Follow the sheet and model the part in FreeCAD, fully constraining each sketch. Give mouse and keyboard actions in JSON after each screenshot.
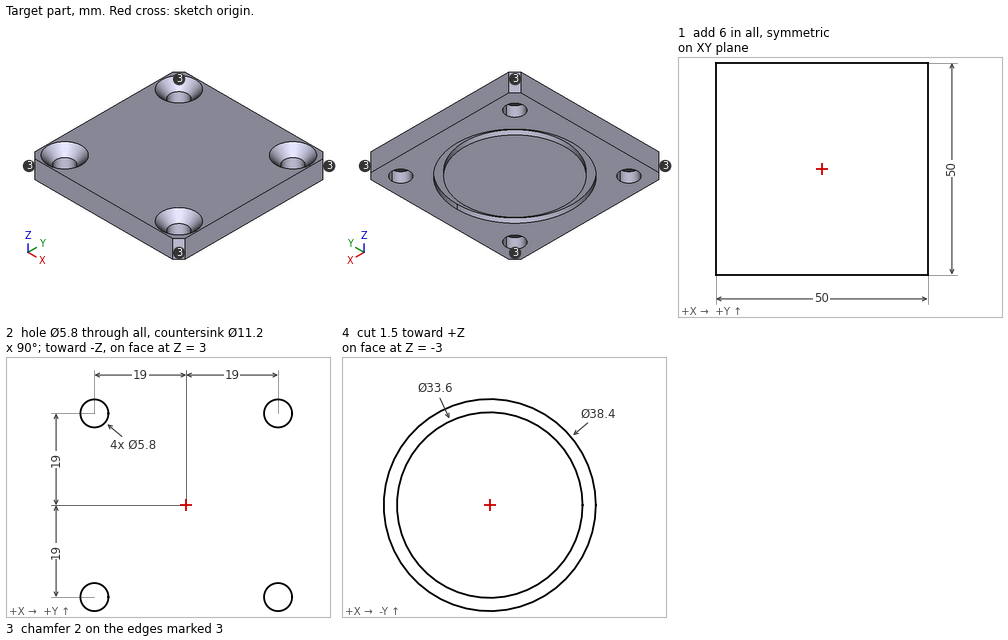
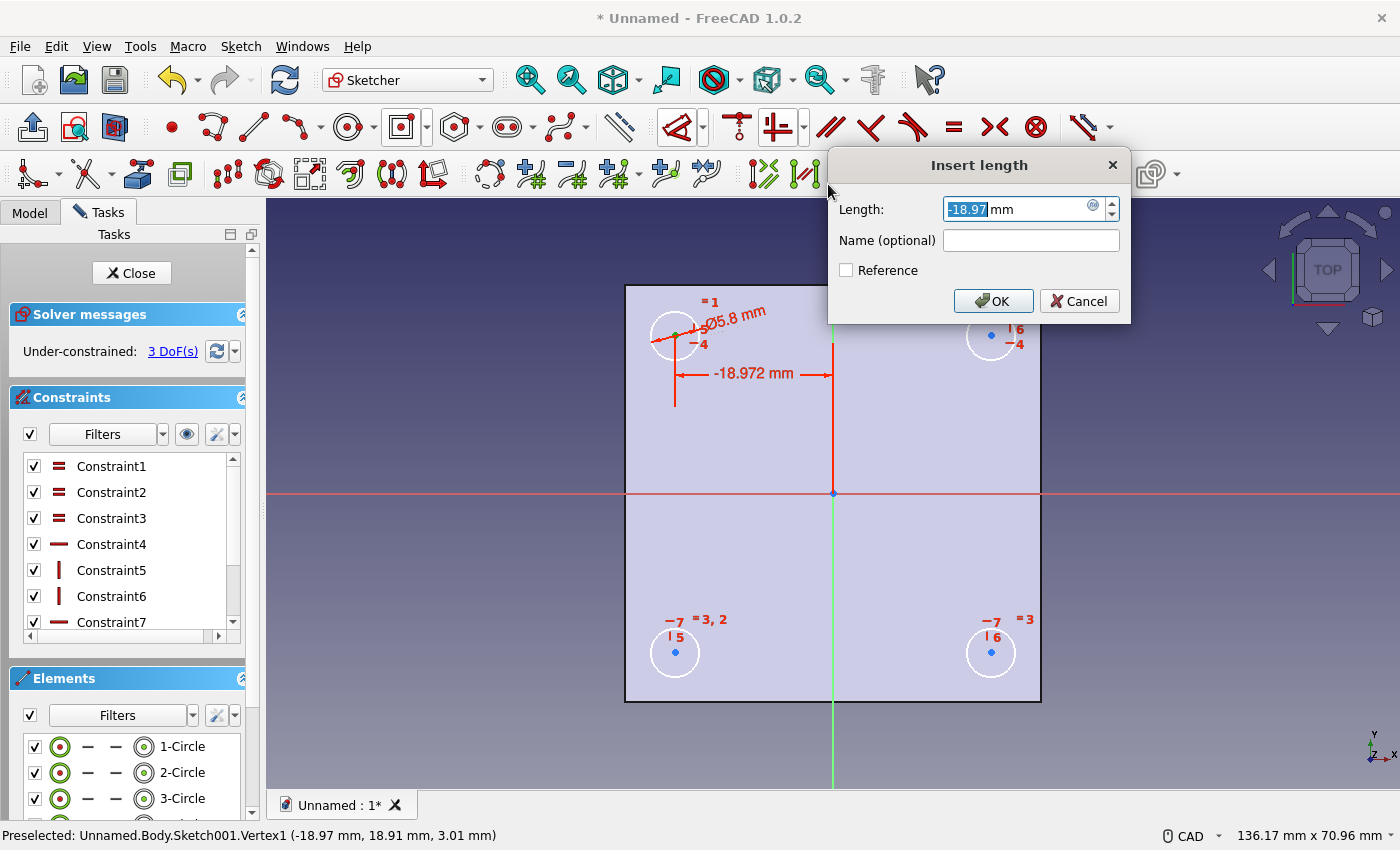
{"action": "type", "text": "-19"}
{"action": "key", "text": "Return"}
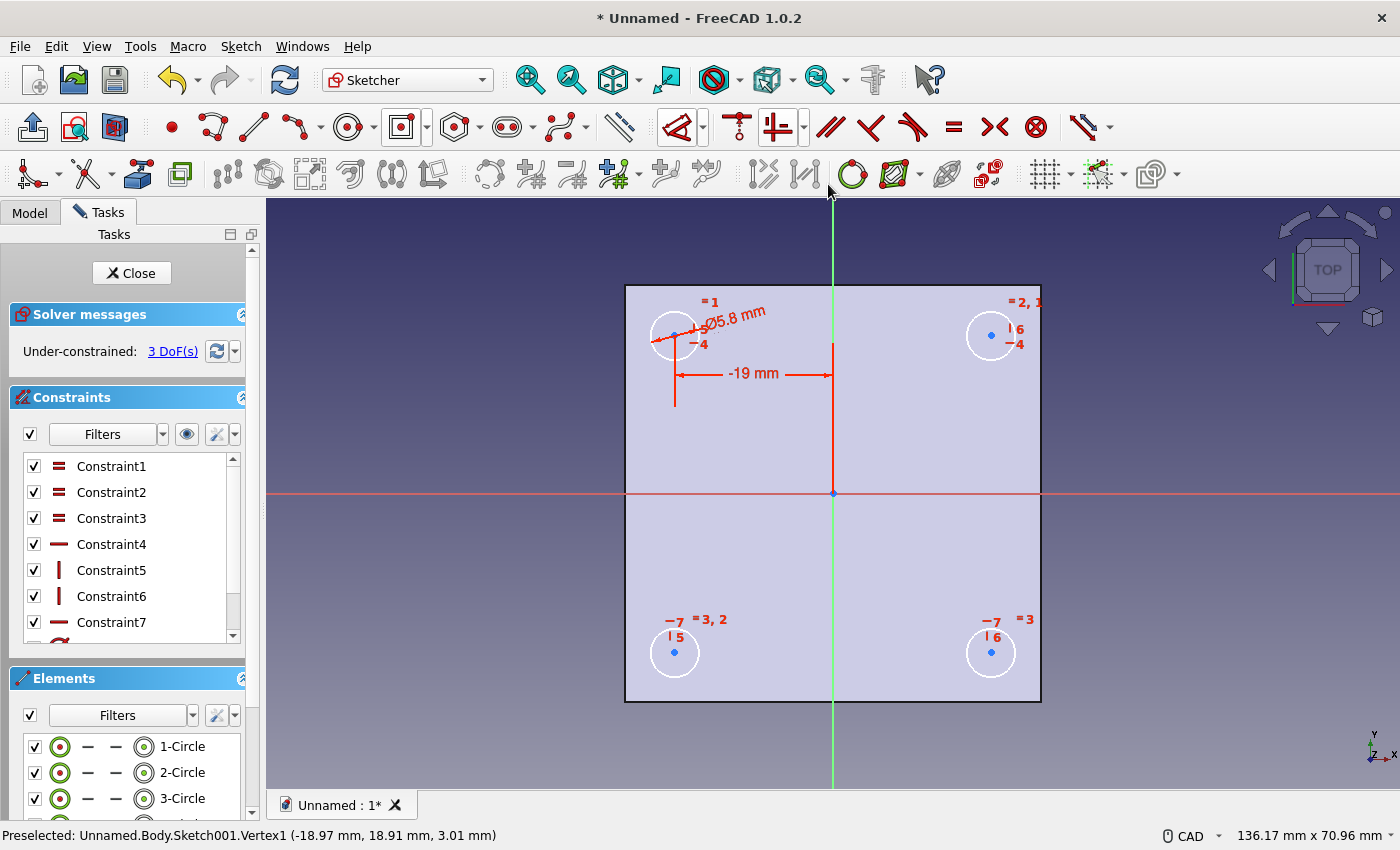
{"action": "left_click", "coordinate": [675, 336]}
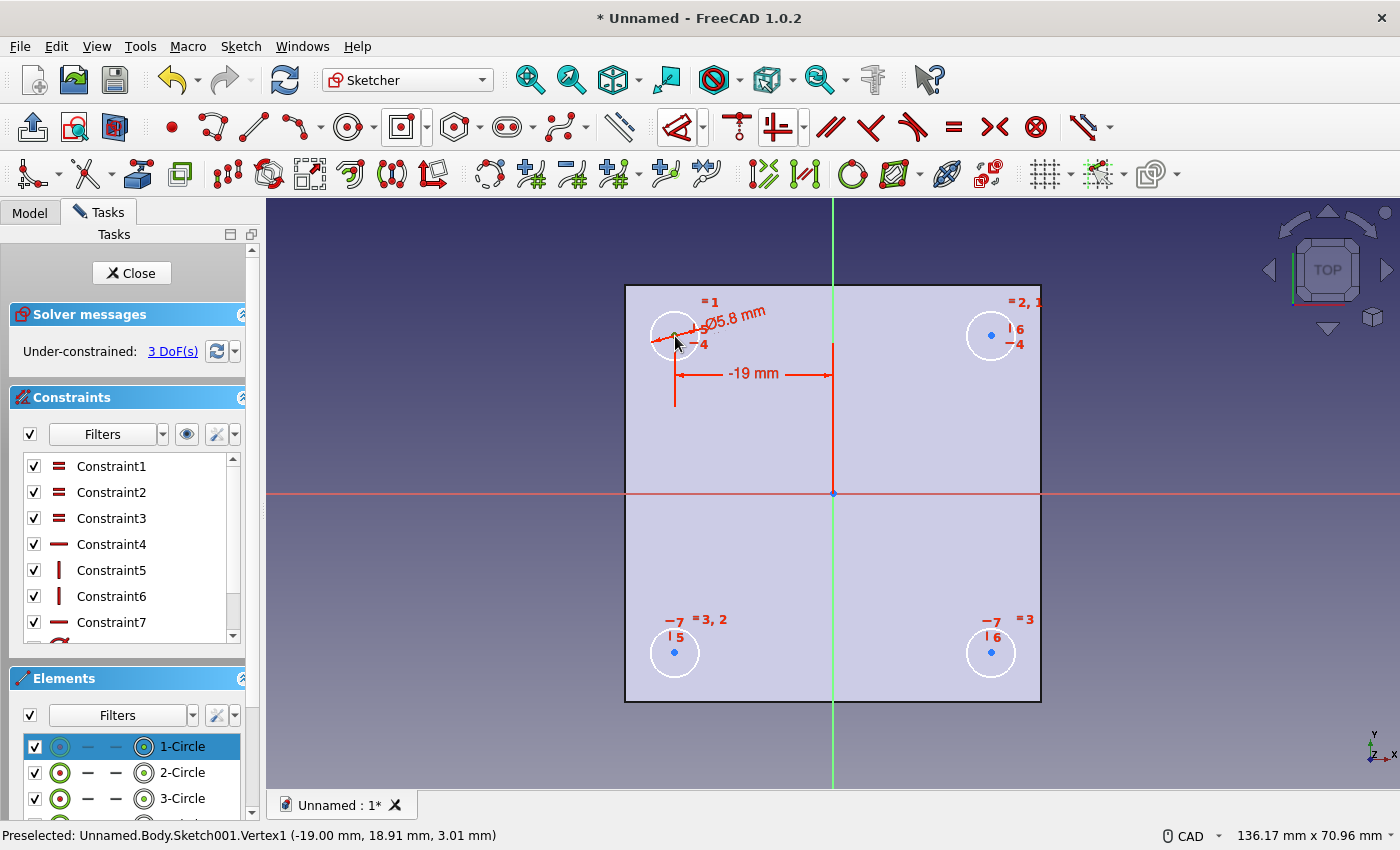
{"action": "key", "text": "i"}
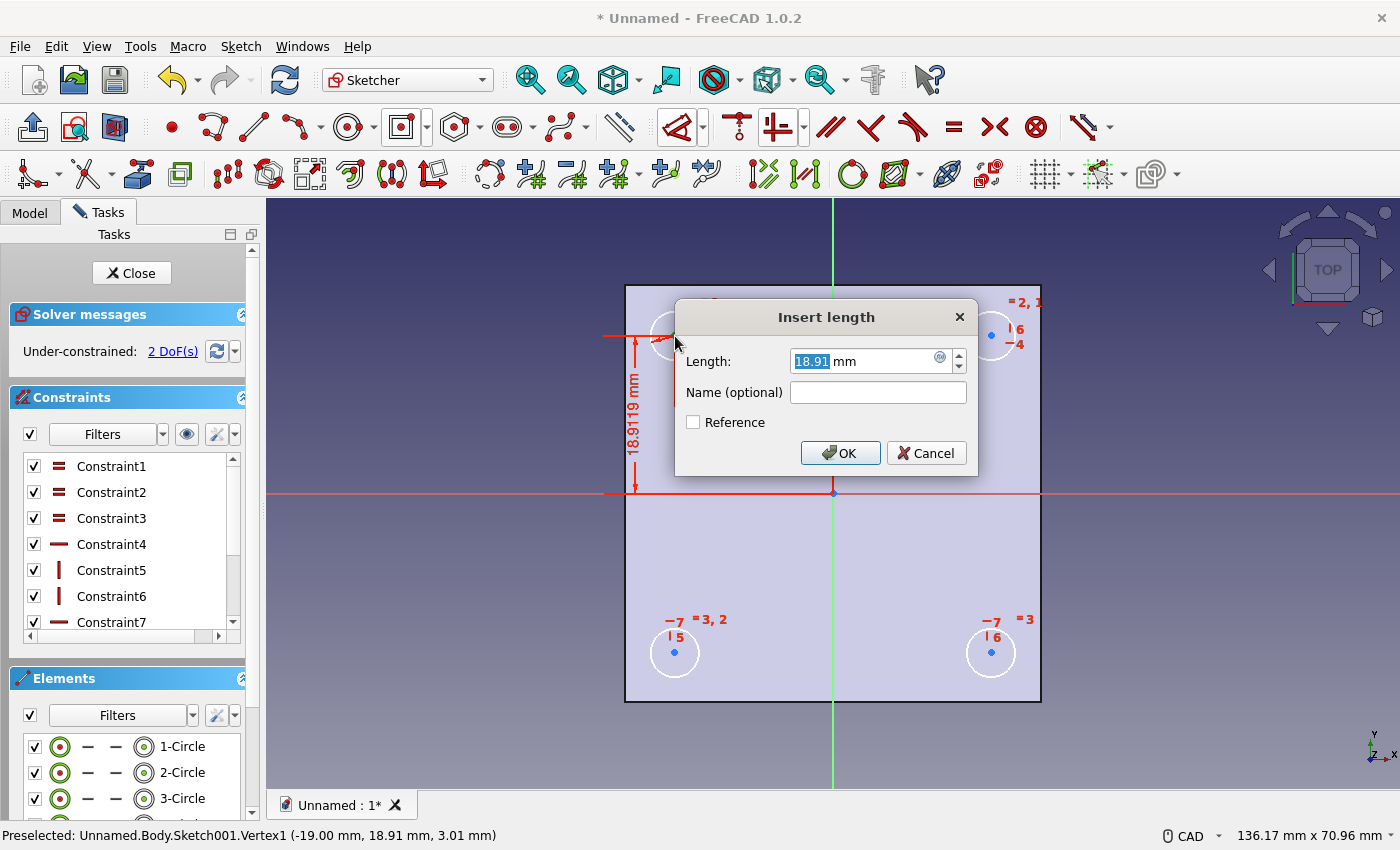
{"action": "type", "text": "19"}
{"action": "key", "text": "Return"}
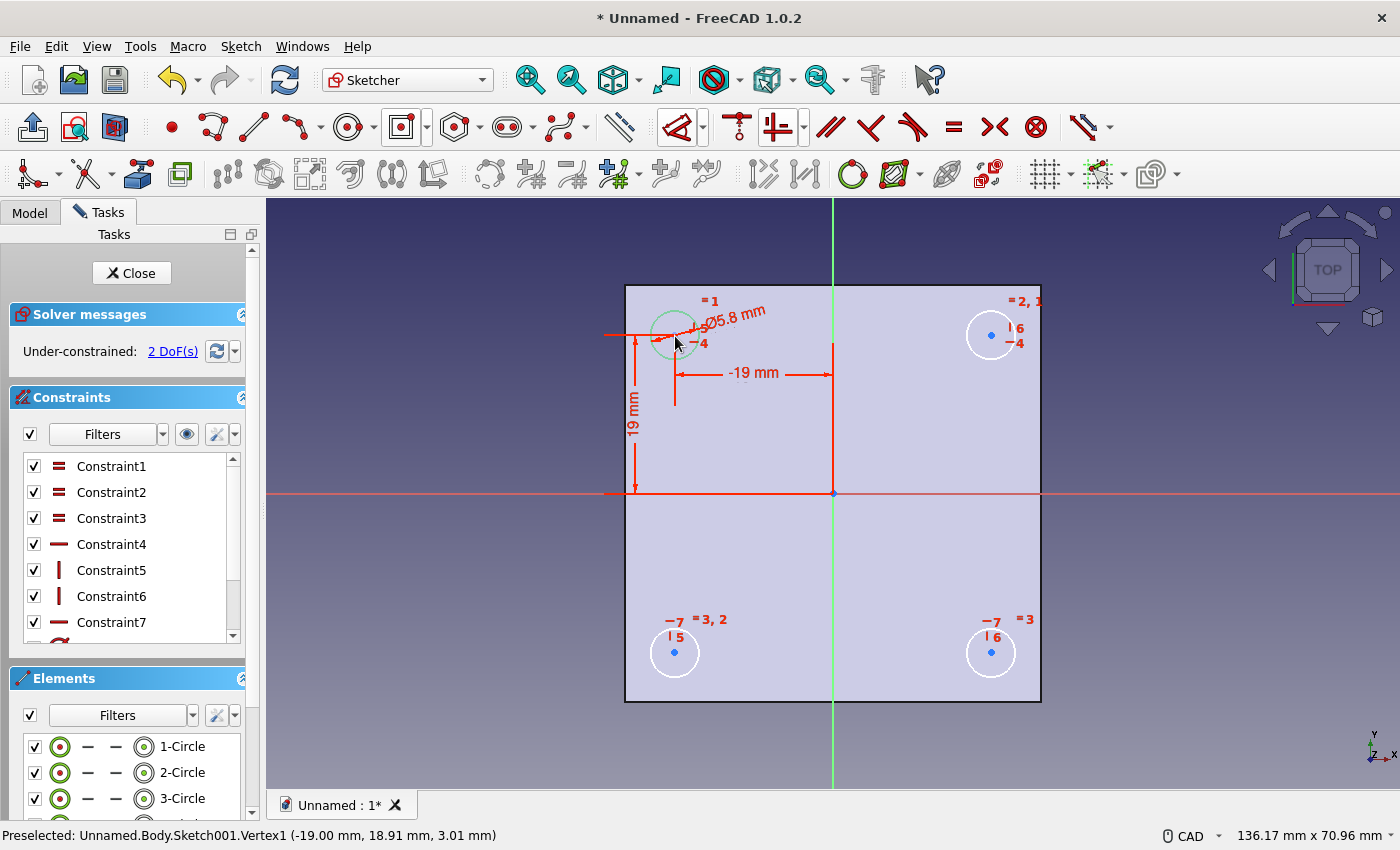
{"action": "left_click", "coordinate": [991, 335]}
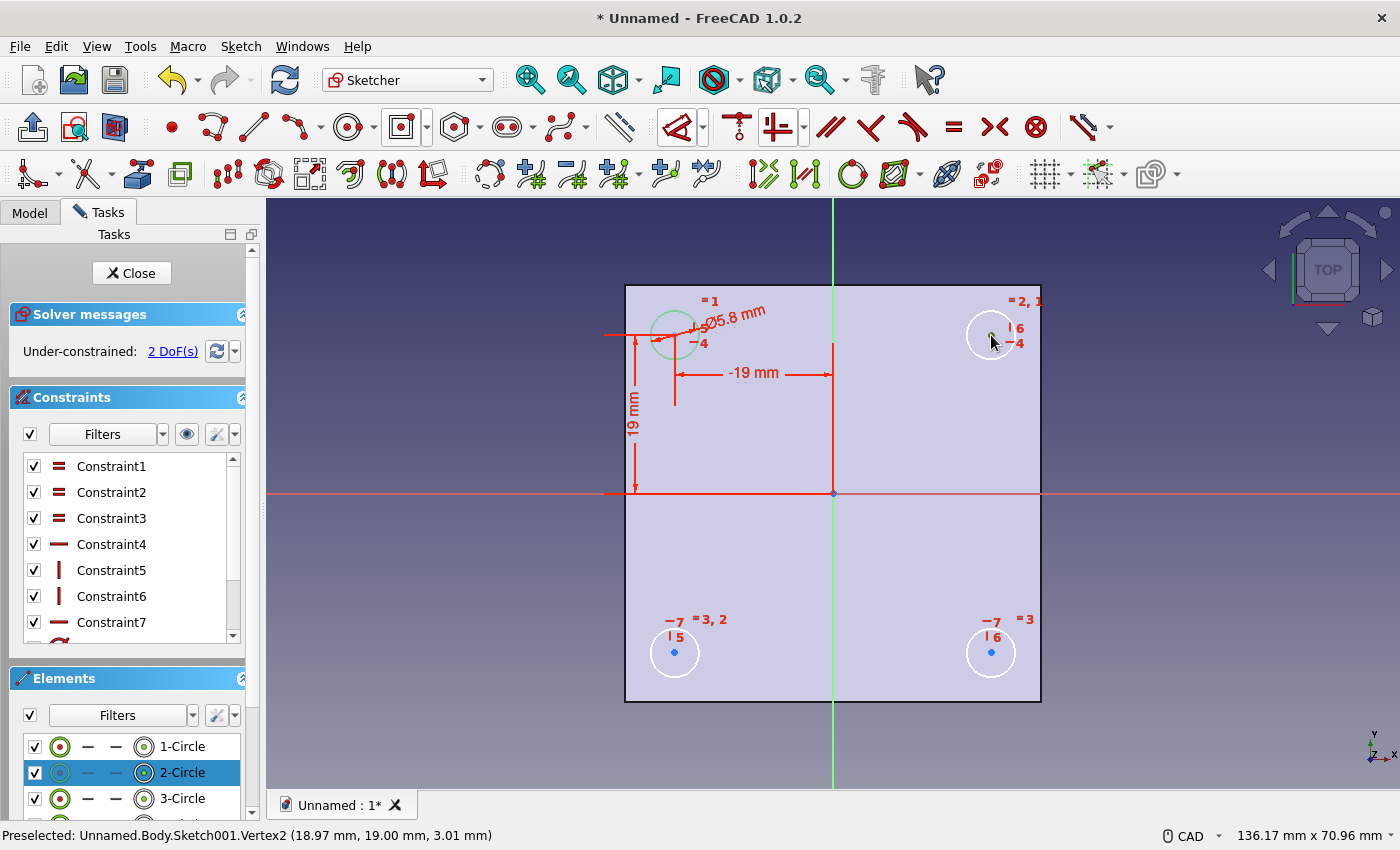
{"action": "left_click", "coordinate": [702, 128]}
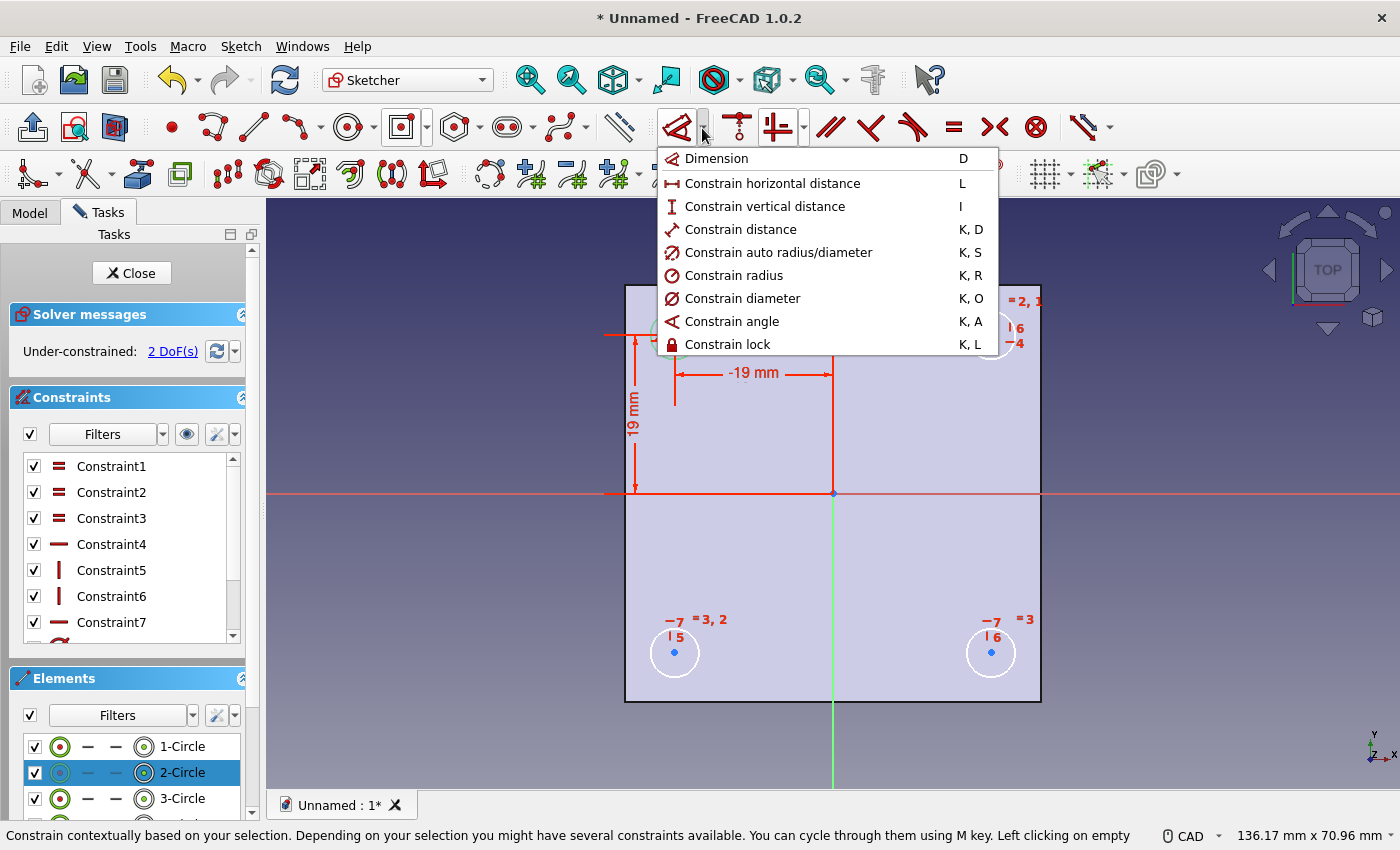
{"action": "left_click", "coordinate": [828, 184]}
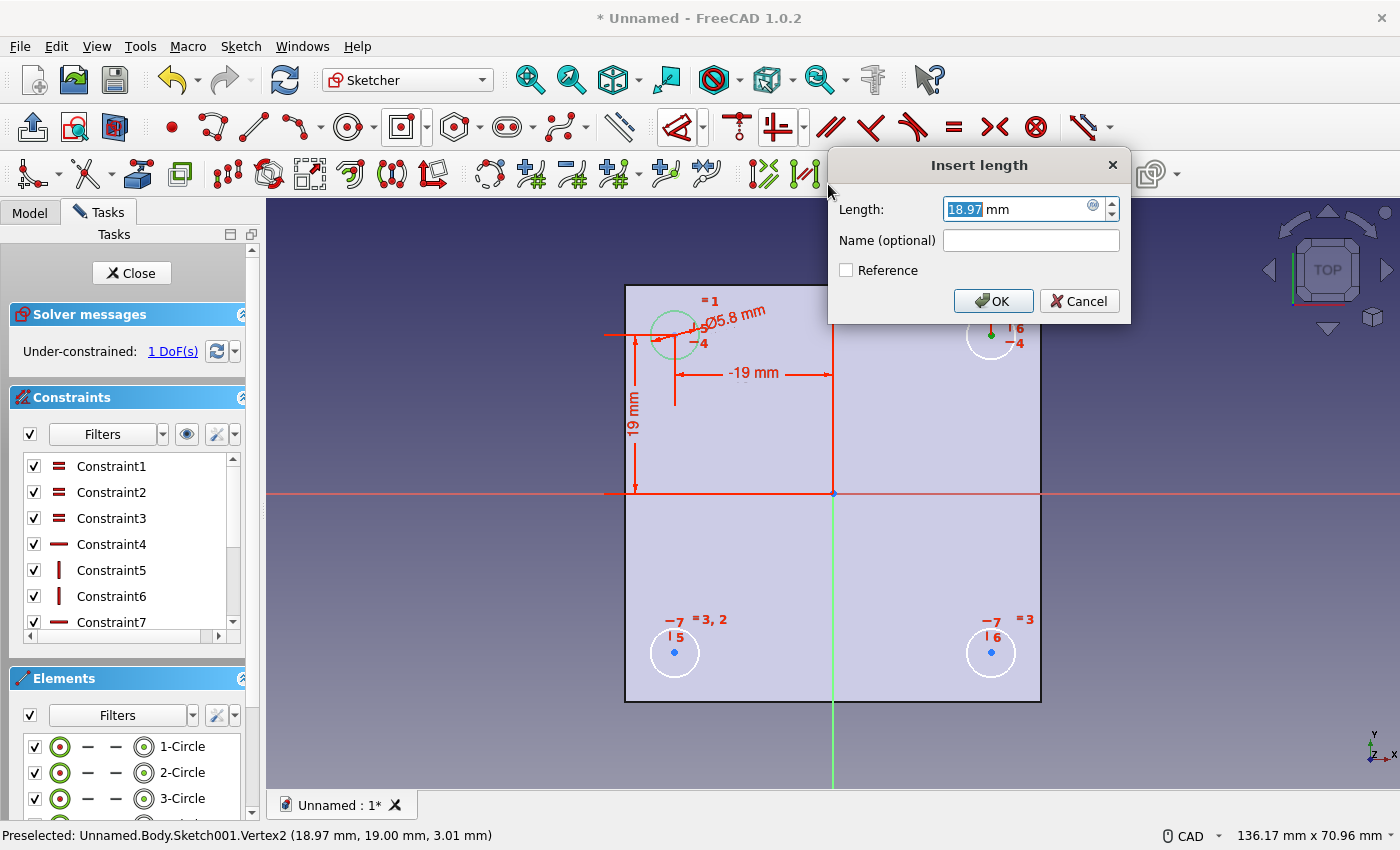
{"action": "type", "text": "19"}
{"action": "key", "text": "Return"}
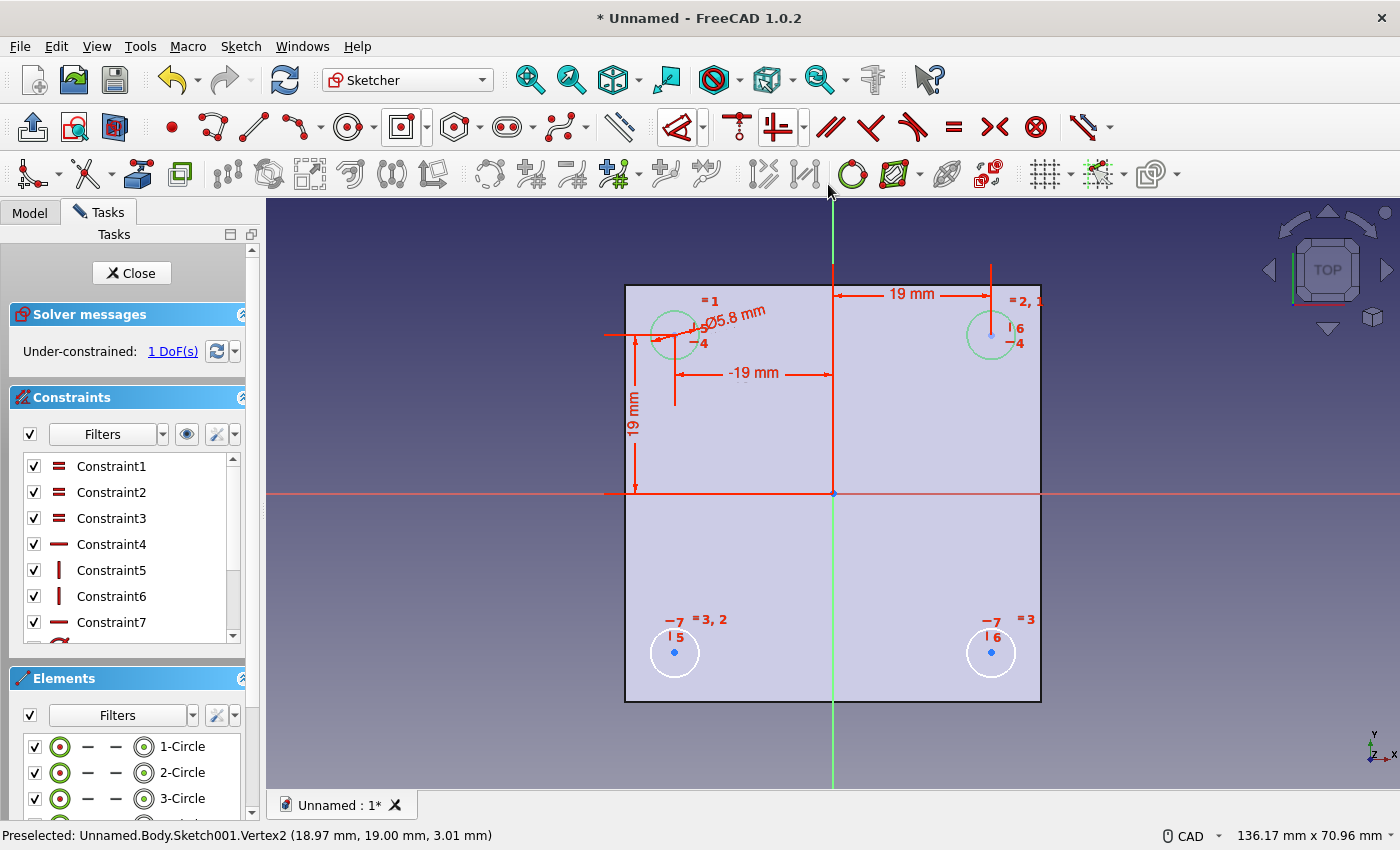
{"action": "left_click", "coordinate": [675, 653]}